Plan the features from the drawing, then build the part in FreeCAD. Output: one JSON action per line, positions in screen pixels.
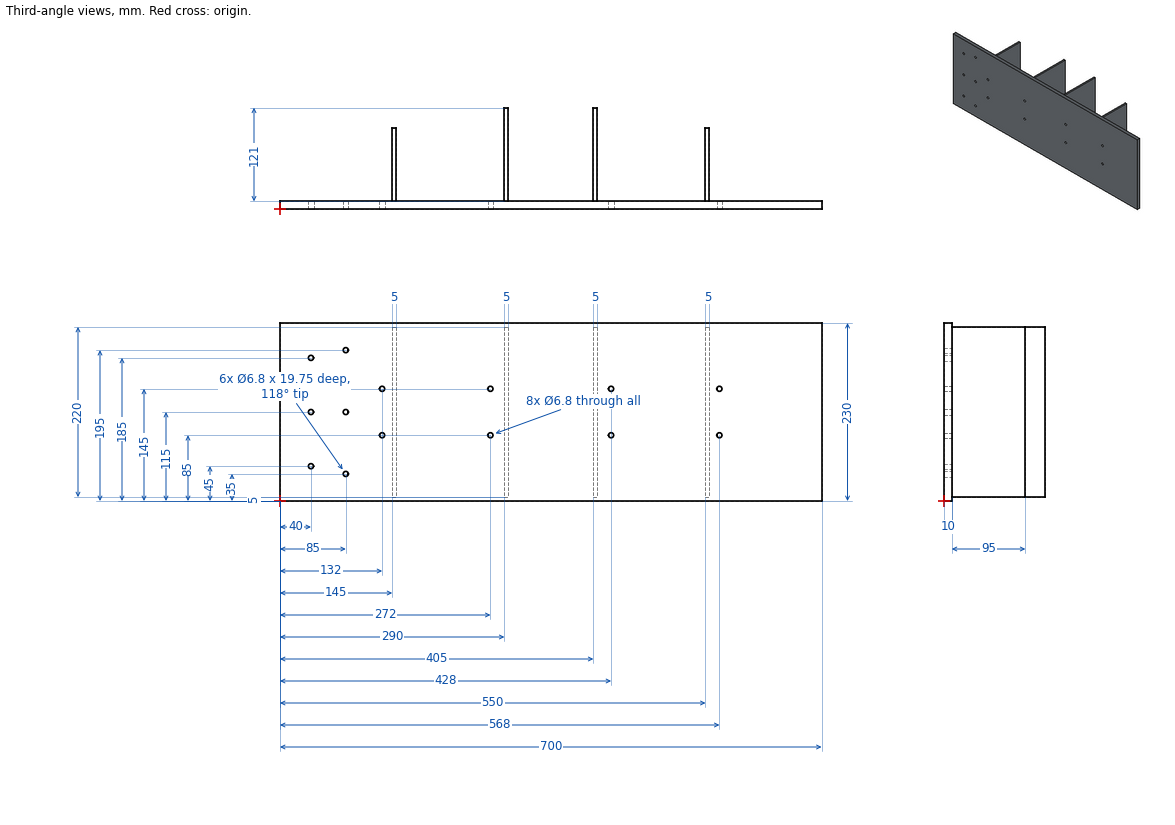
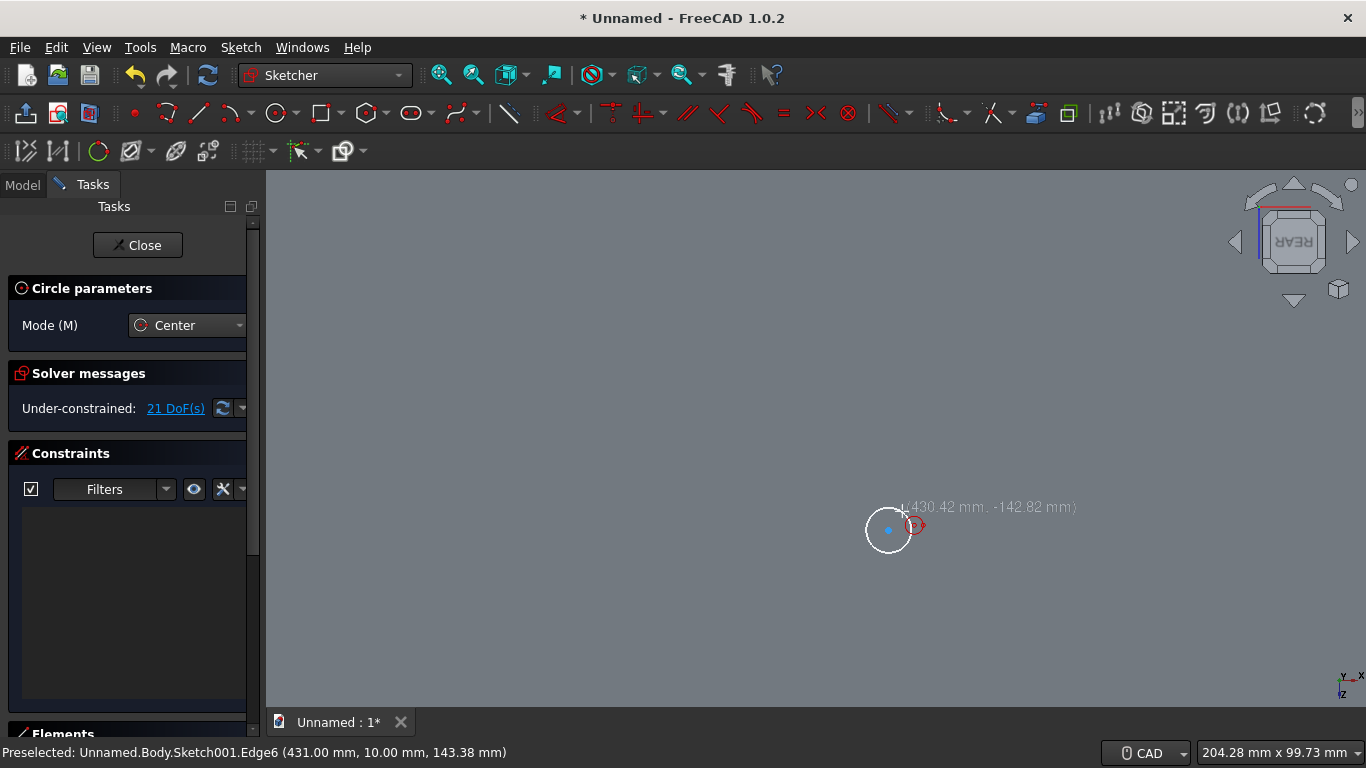
{"action": "scroll", "coordinate": [889, 201], "scroll_direction": "up", "scroll_amount": 2}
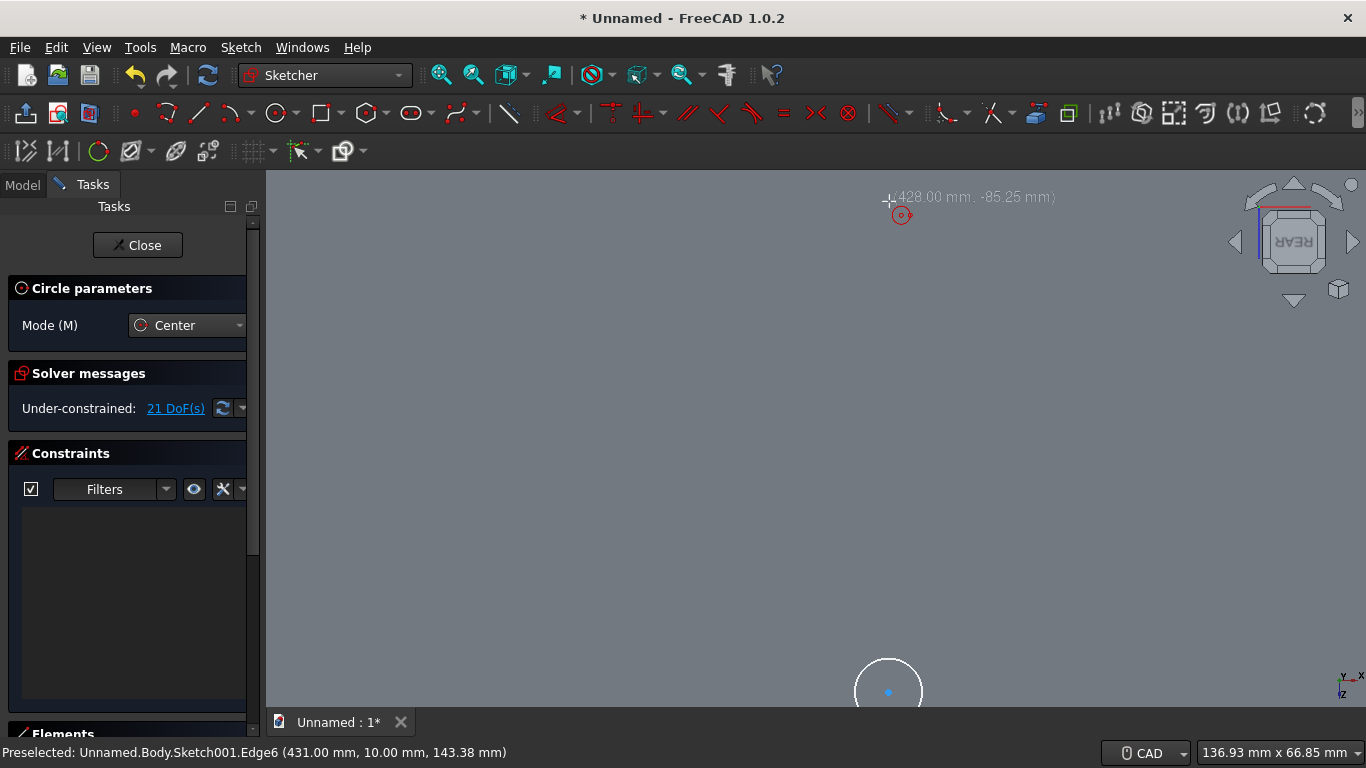
{"action": "scroll", "coordinate": [904, 489], "scroll_direction": "down", "scroll_amount": 10}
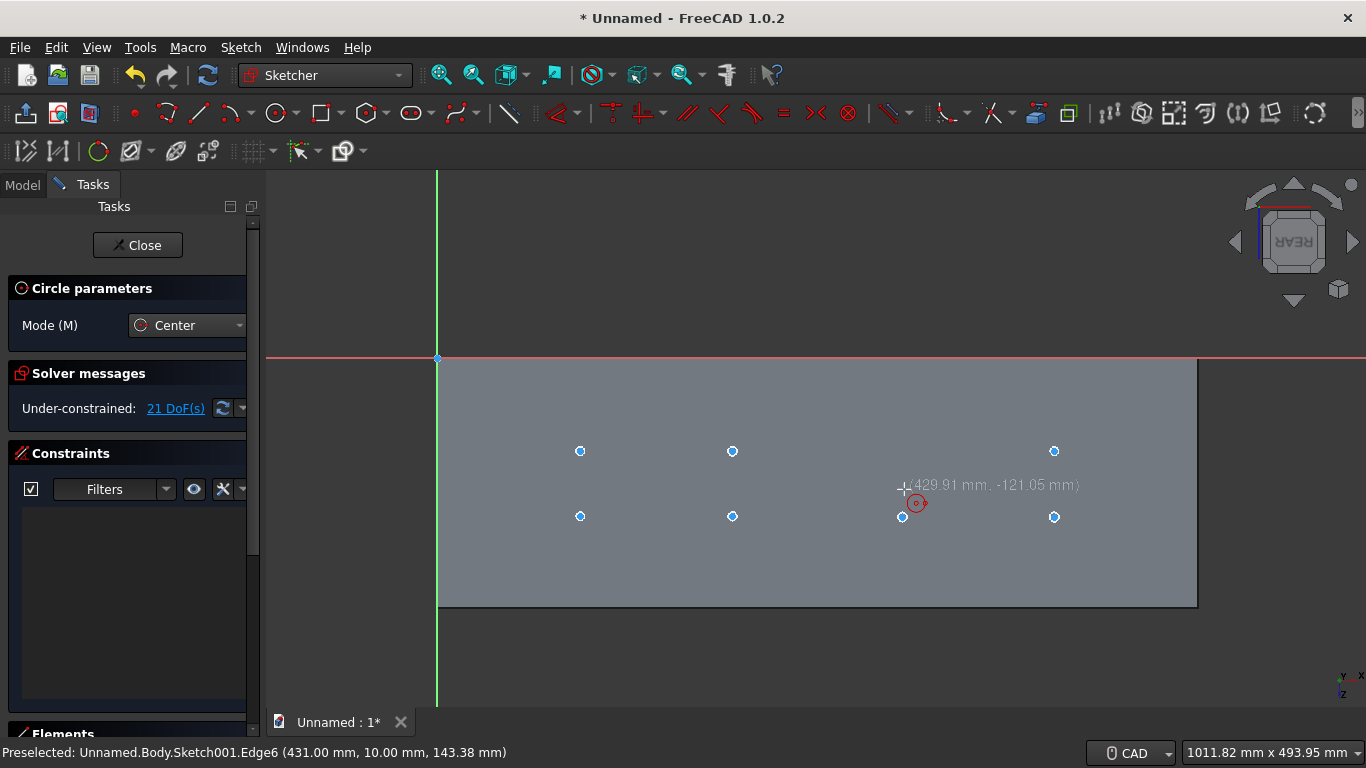
{"action": "left_click", "coordinate": [902, 450]}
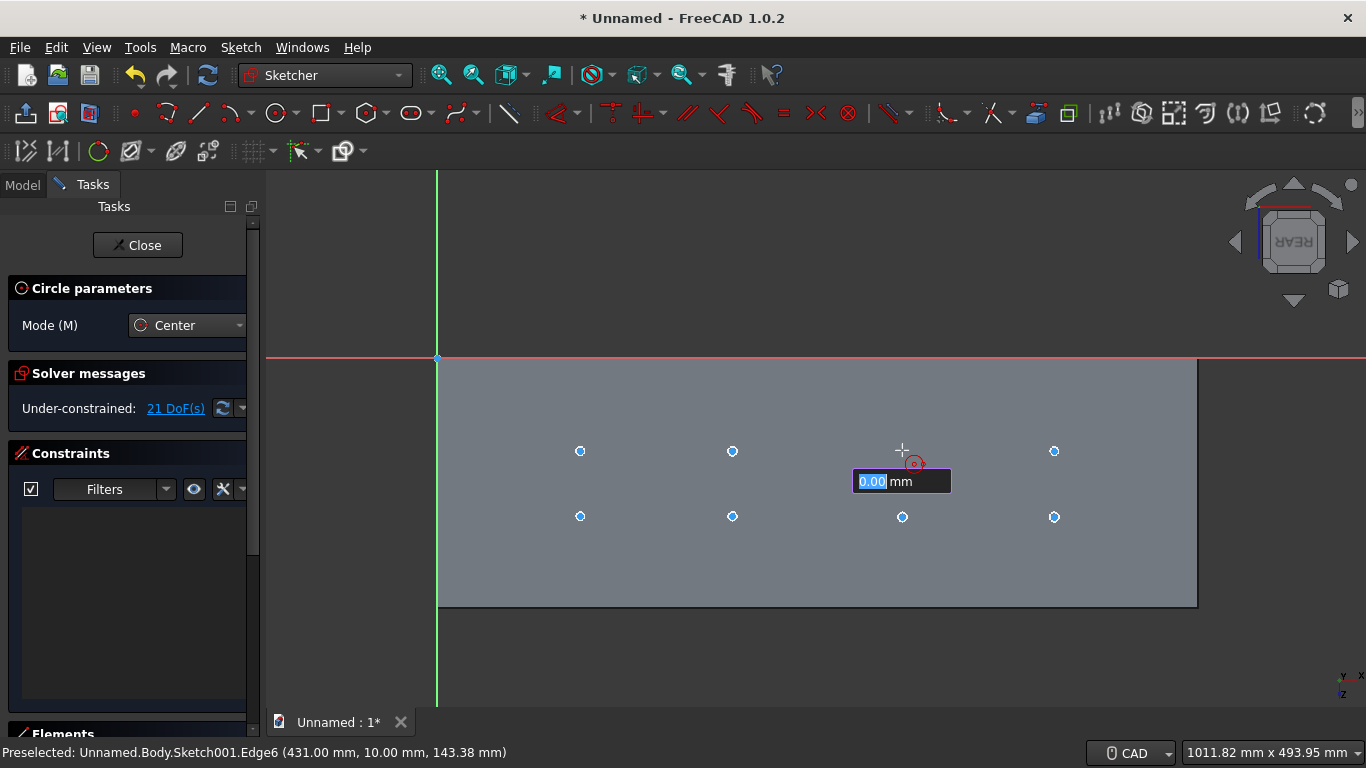
{"action": "scroll", "coordinate": [905, 448], "scroll_direction": "up", "scroll_amount": 8}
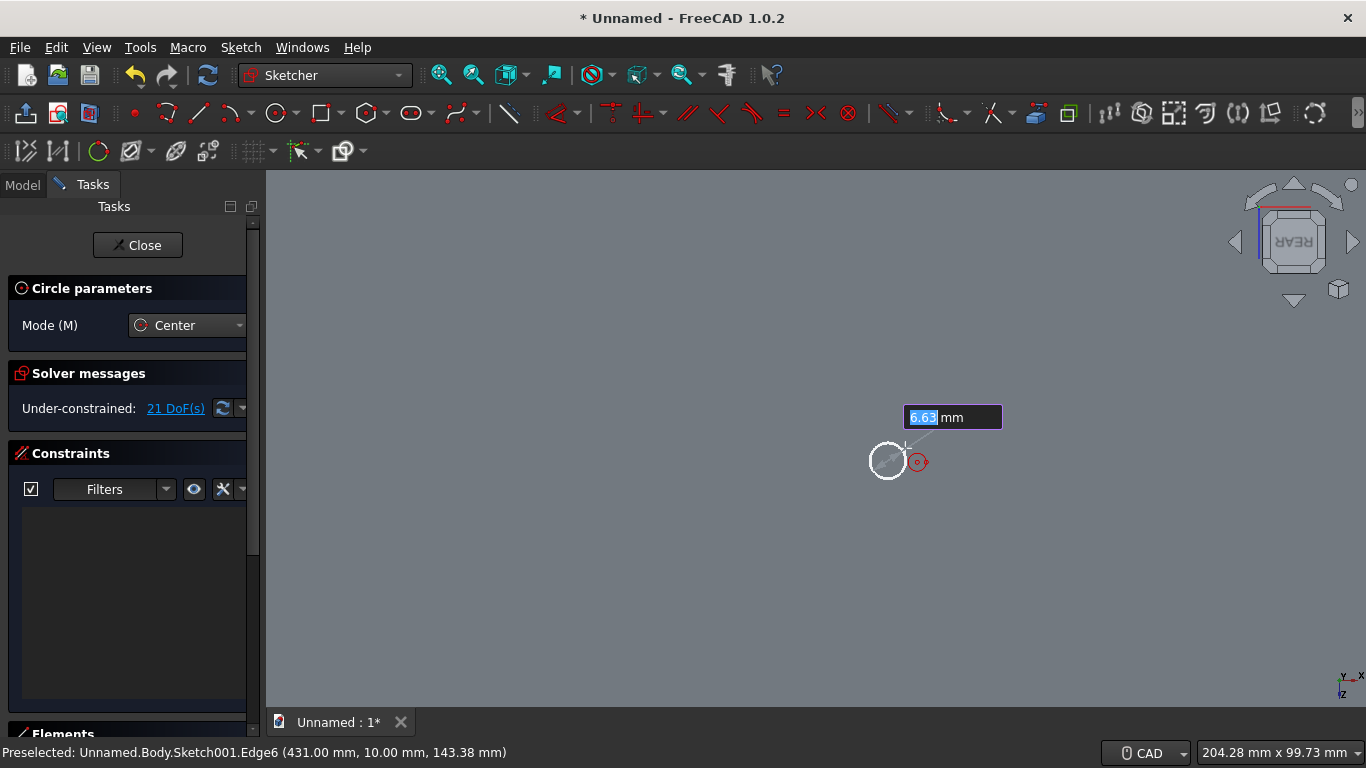
{"action": "left_click", "coordinate": [903, 445]}
{"action": "key", "text": "Escape"}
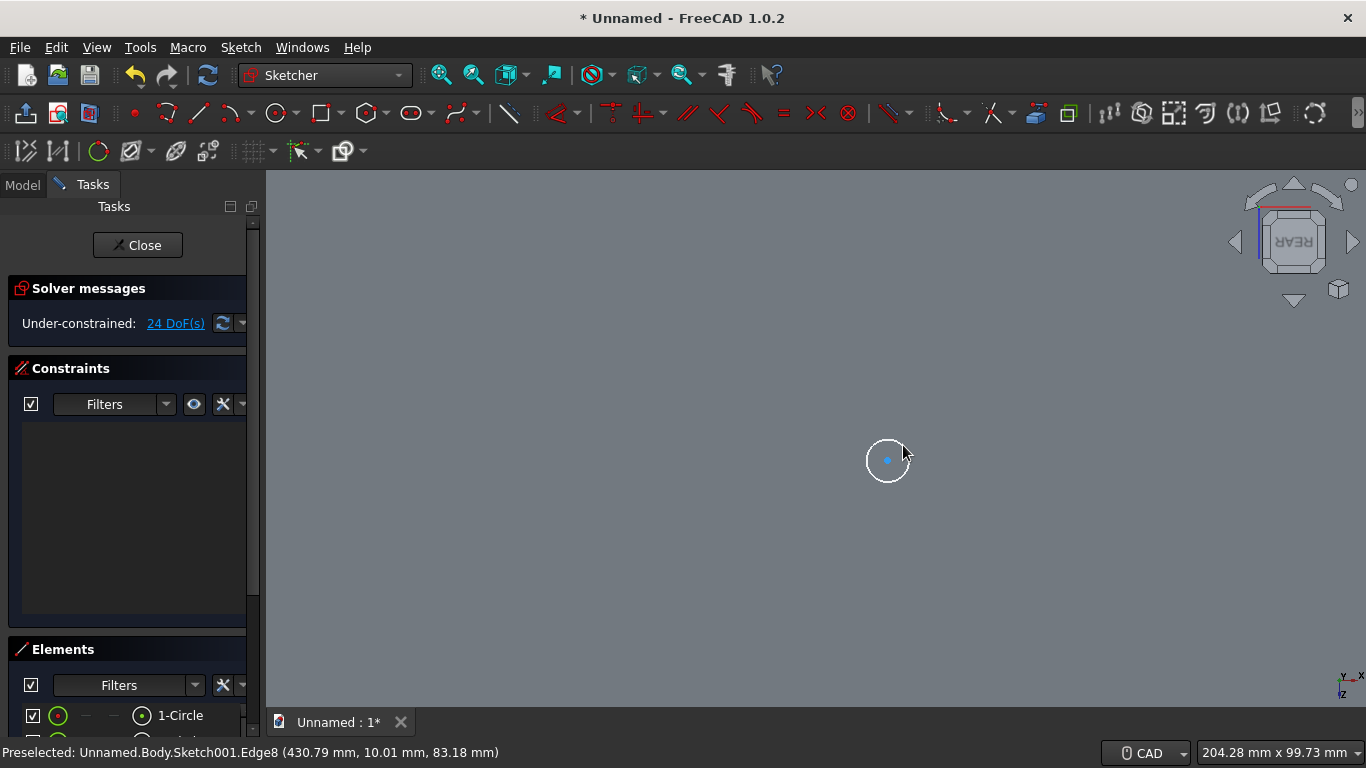
{"action": "scroll", "coordinate": [905, 448], "scroll_direction": "down", "scroll_amount": 8}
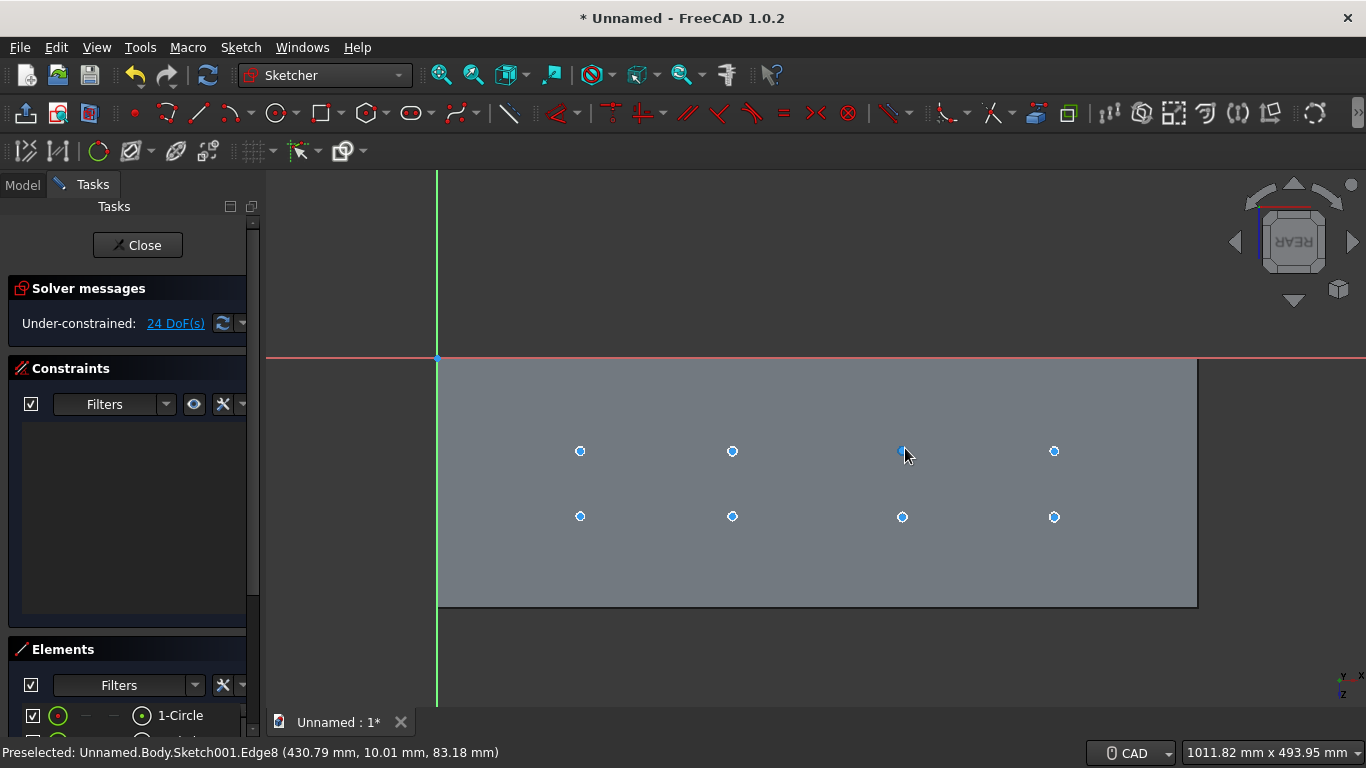
{"action": "scroll", "coordinate": [736, 448], "scroll_direction": "up", "scroll_amount": 6}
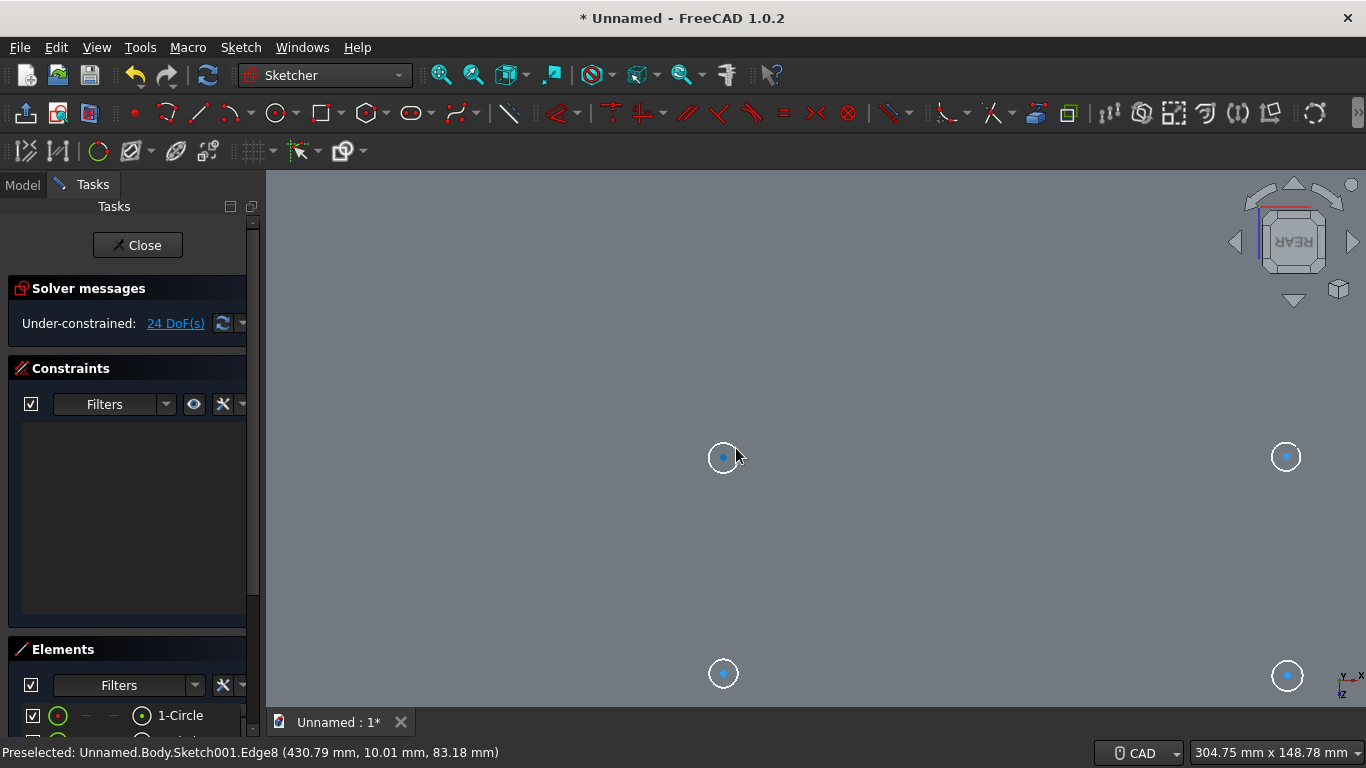
{"action": "left_click", "coordinate": [734, 447]}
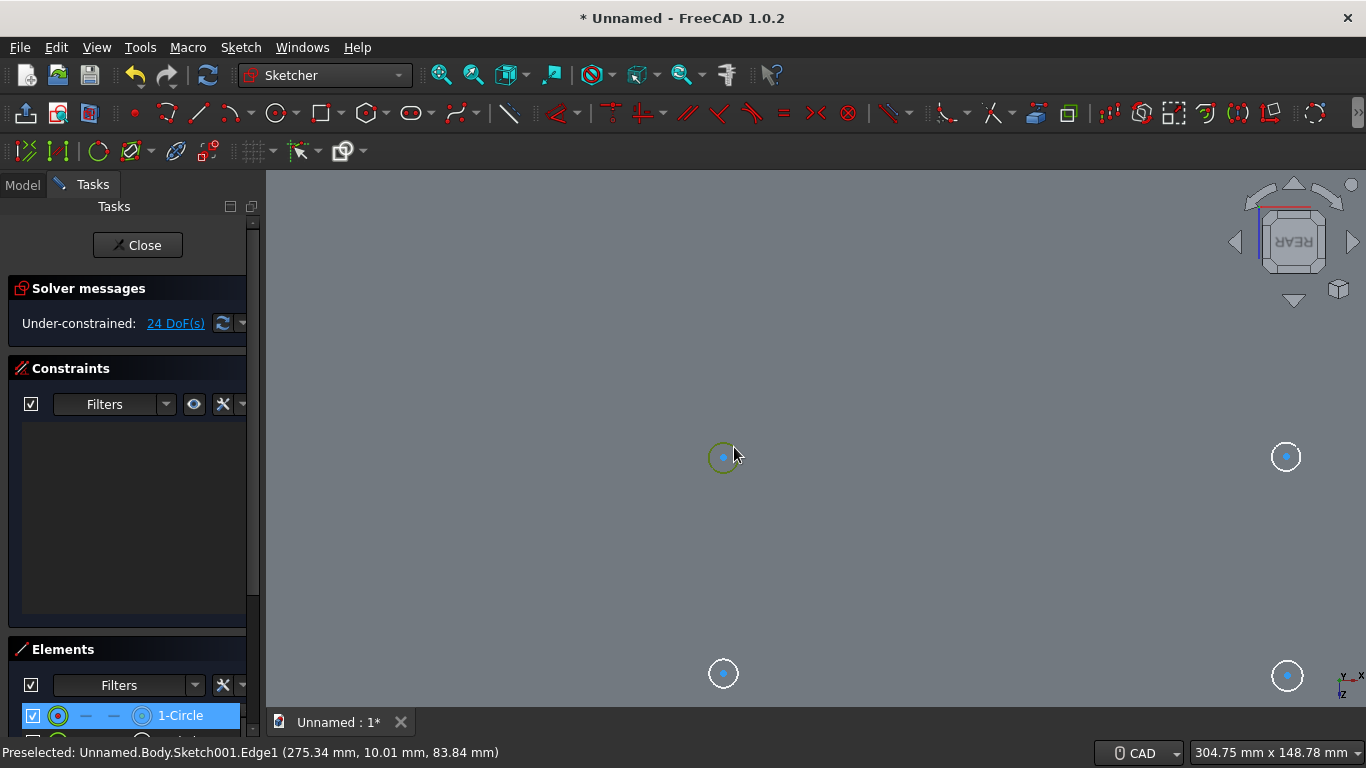
{"action": "left_click", "coordinate": [733, 664]}